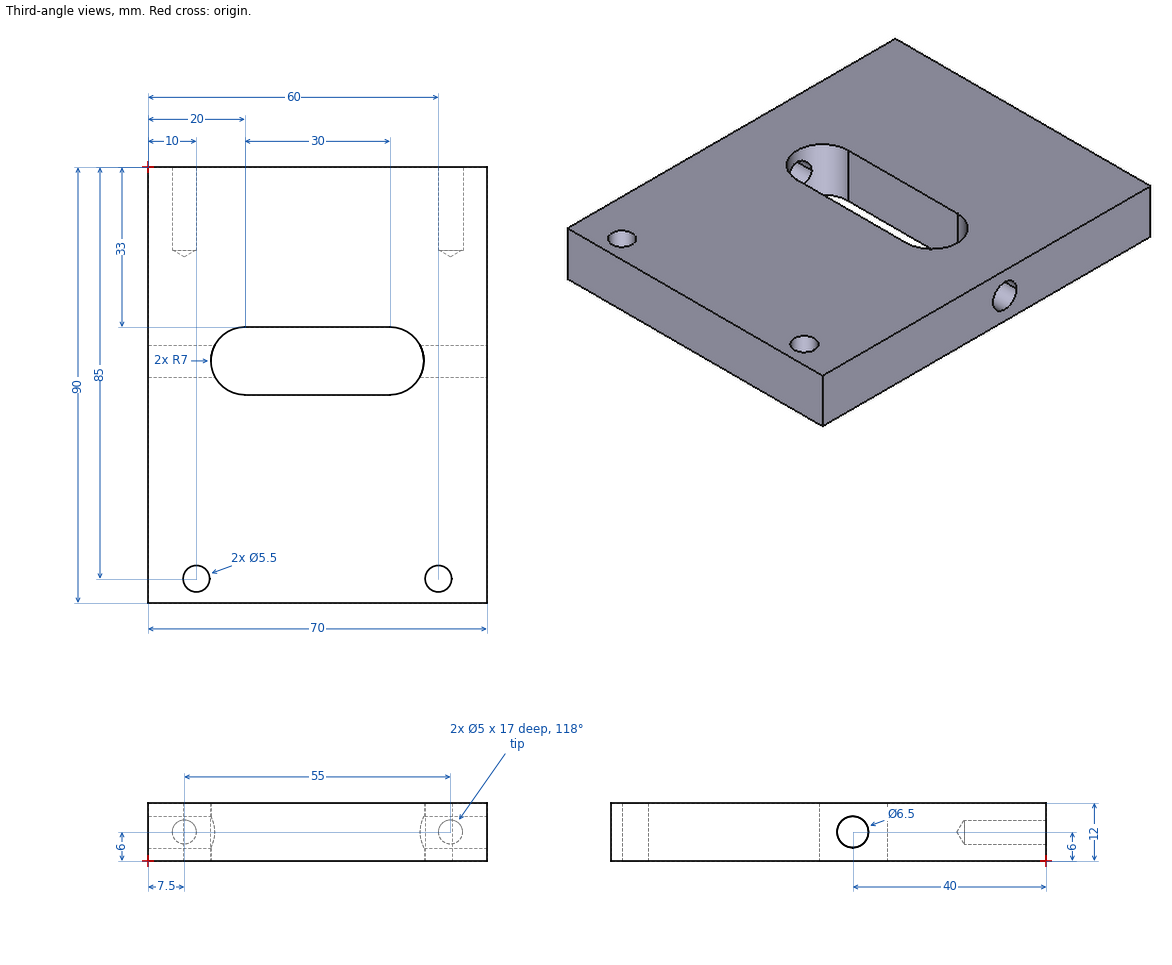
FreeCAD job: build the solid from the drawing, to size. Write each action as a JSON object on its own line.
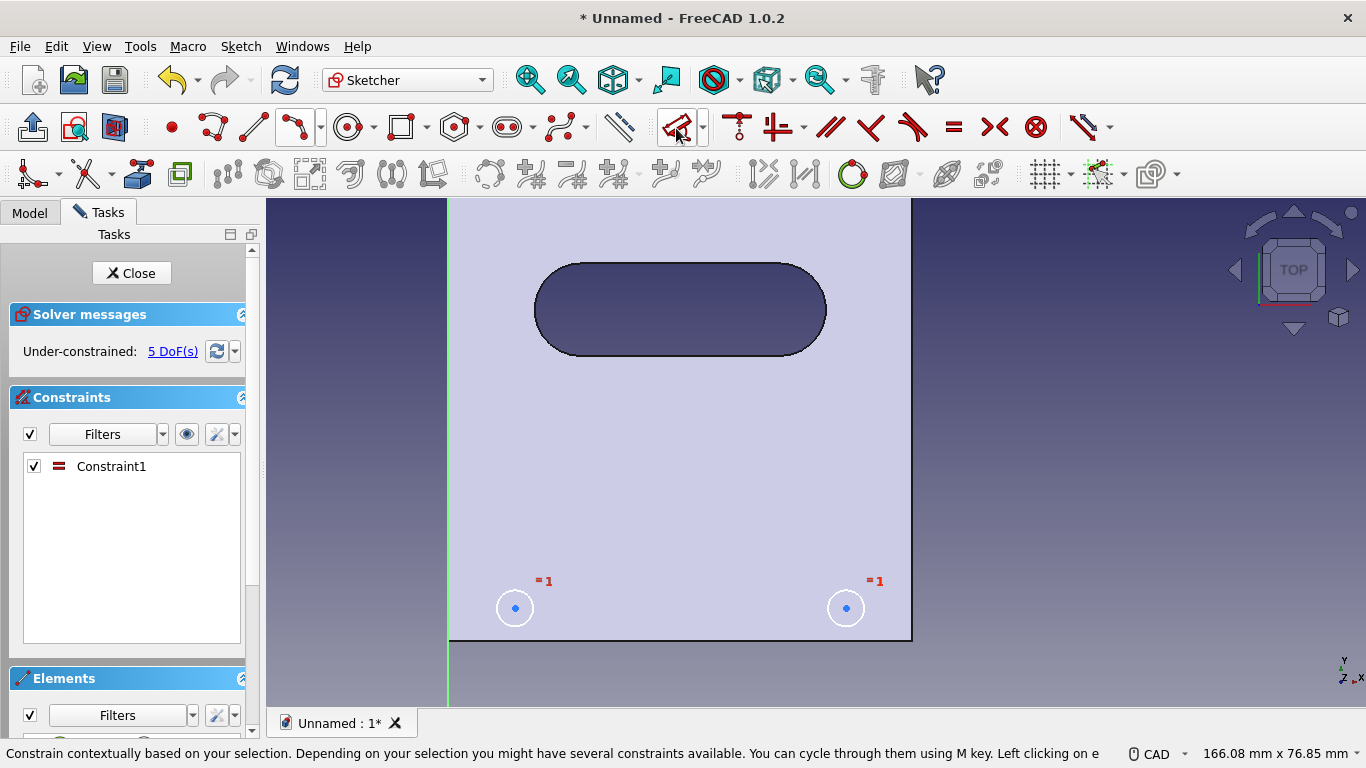
{"action": "left_click", "coordinate": [528, 596]}
{"action": "left_click", "coordinate": [551, 574]}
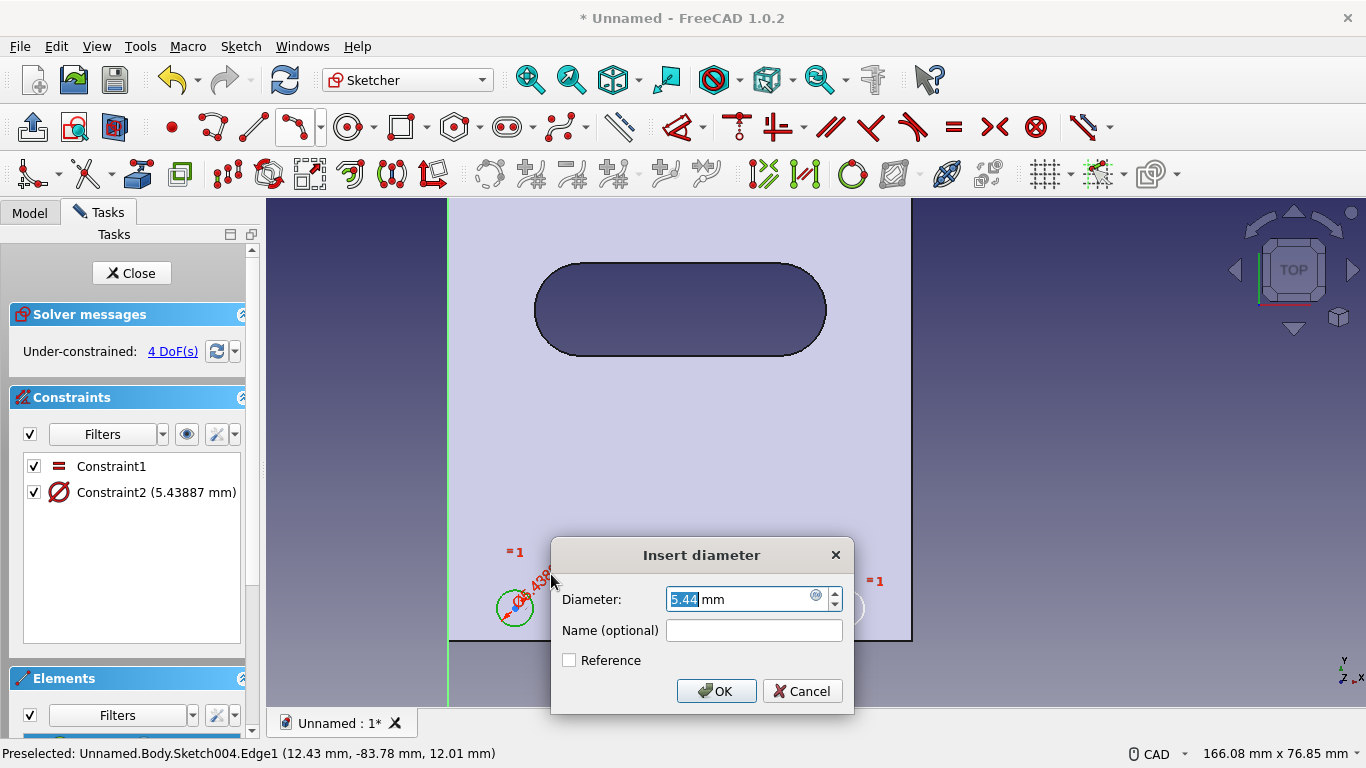
{"action": "type", "text": "5.5"}
{"action": "key", "text": "Return"}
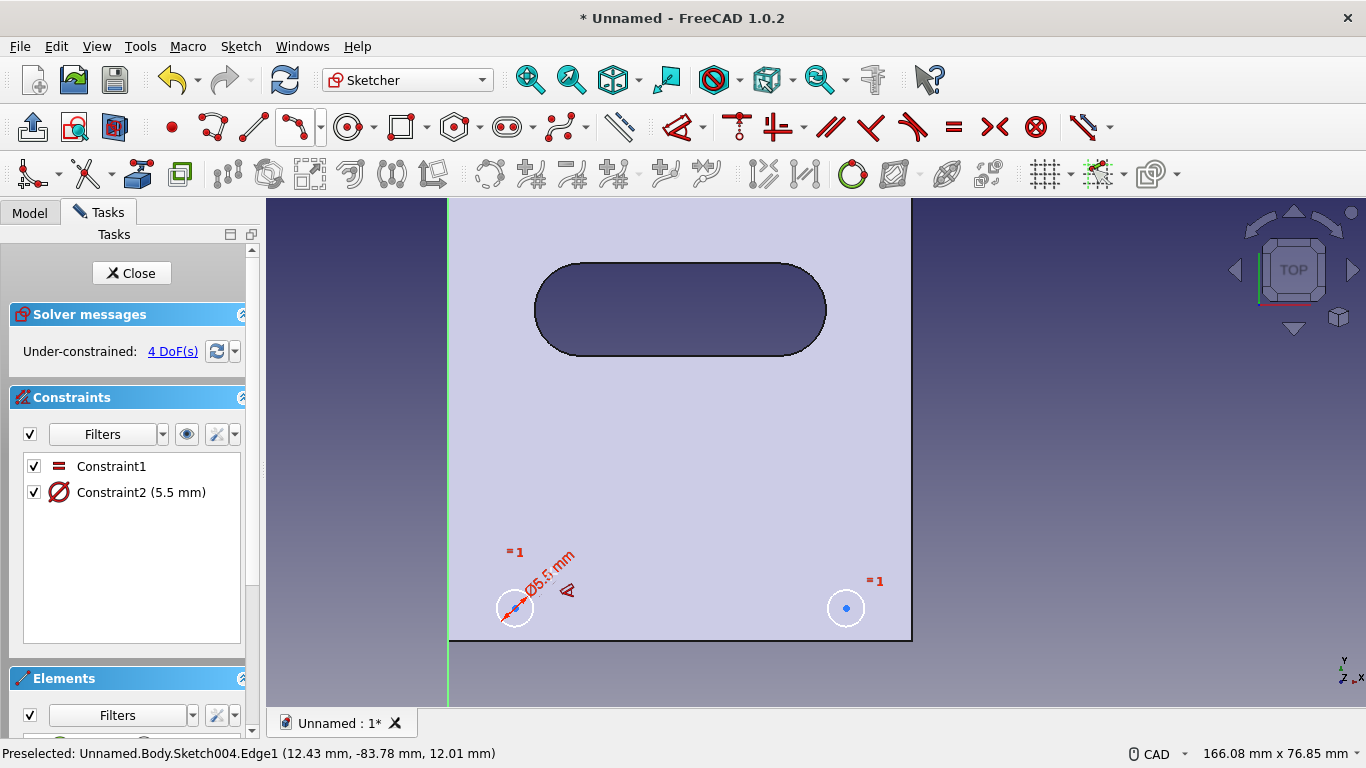
{"action": "left_click", "coordinate": [515, 608]}
{"action": "left_click", "coordinate": [482, 642]}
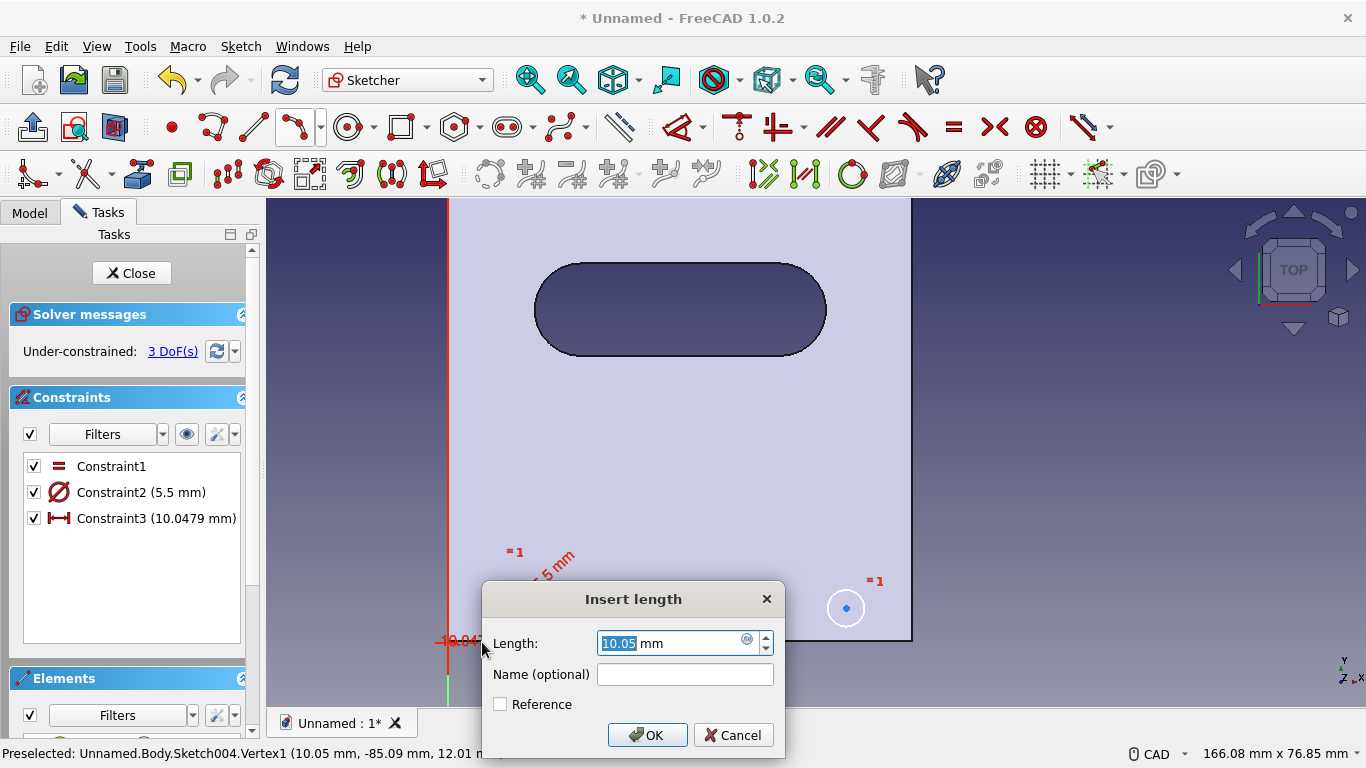
{"action": "type", "text": "10"}
{"action": "key", "text": "Return"}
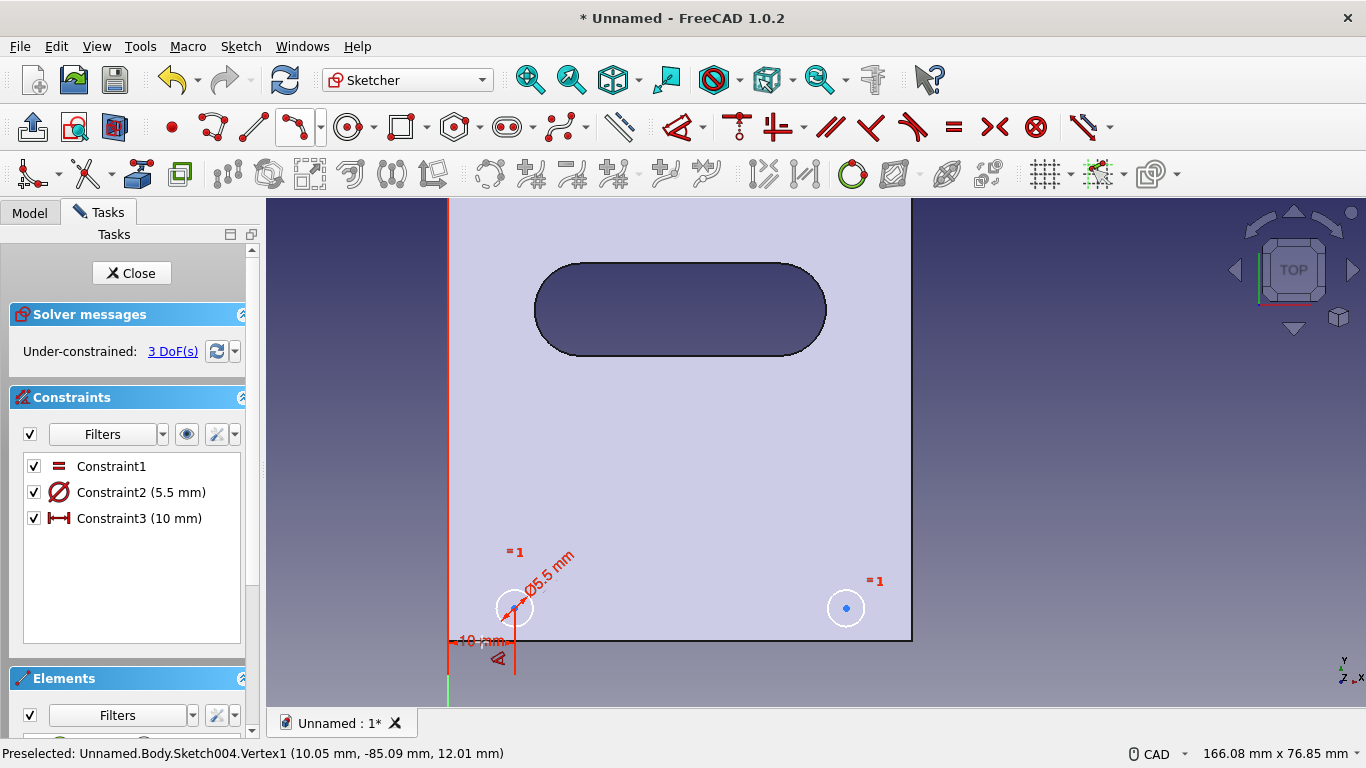
{"action": "left_click", "coordinate": [515, 608]}
{"action": "left_click", "coordinate": [414, 417]}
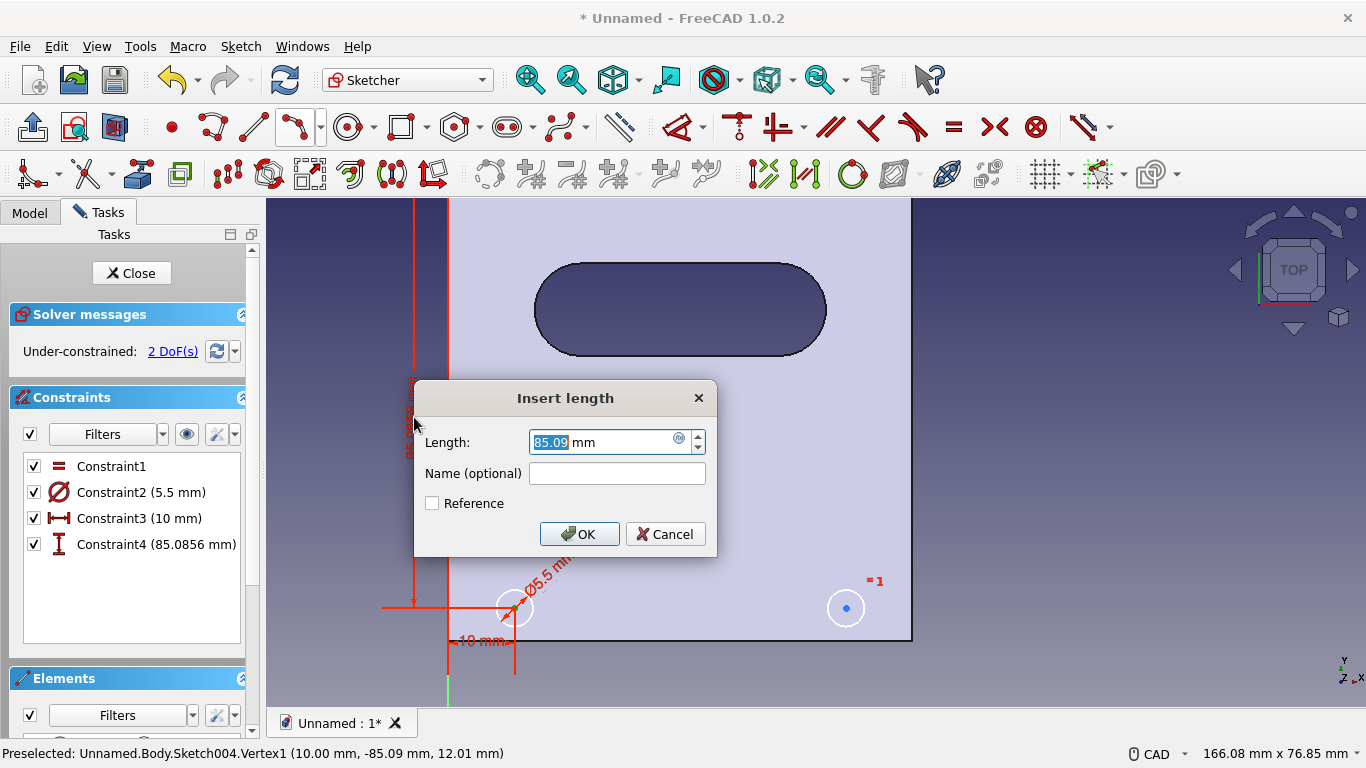
{"action": "type", "text": "85"}
{"action": "key", "text": "Return"}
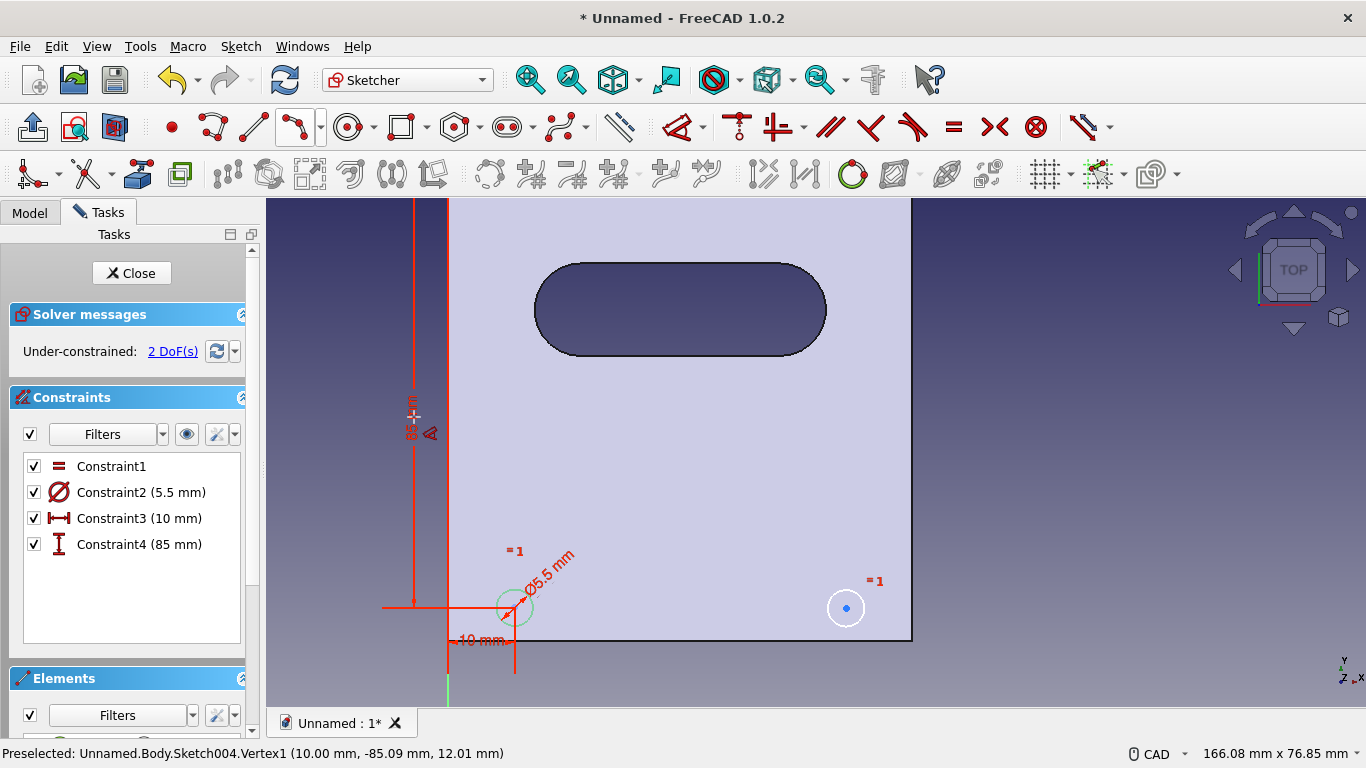
{"action": "left_click", "coordinate": [846, 608]}
{"action": "left_click", "coordinate": [647, 642]}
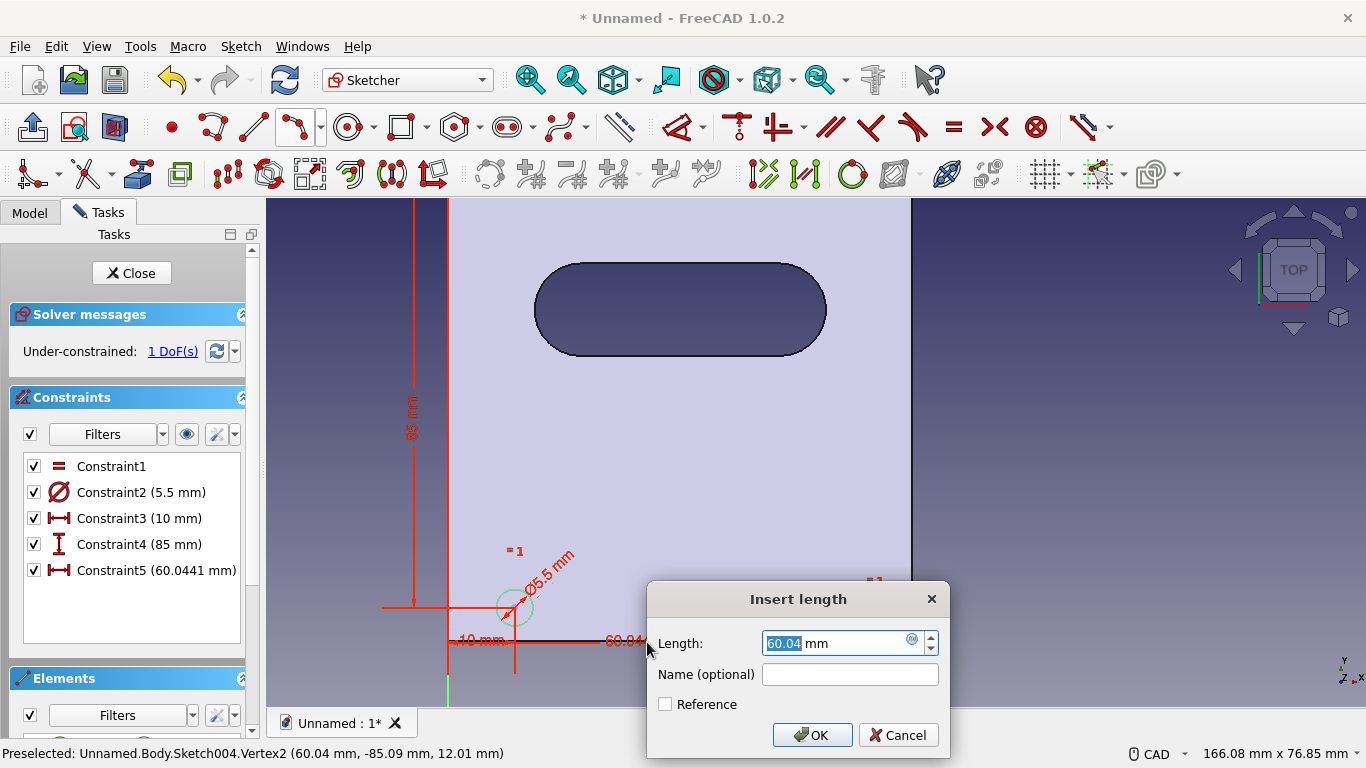
{"action": "type", "text": "60"}
{"action": "key", "text": "Return"}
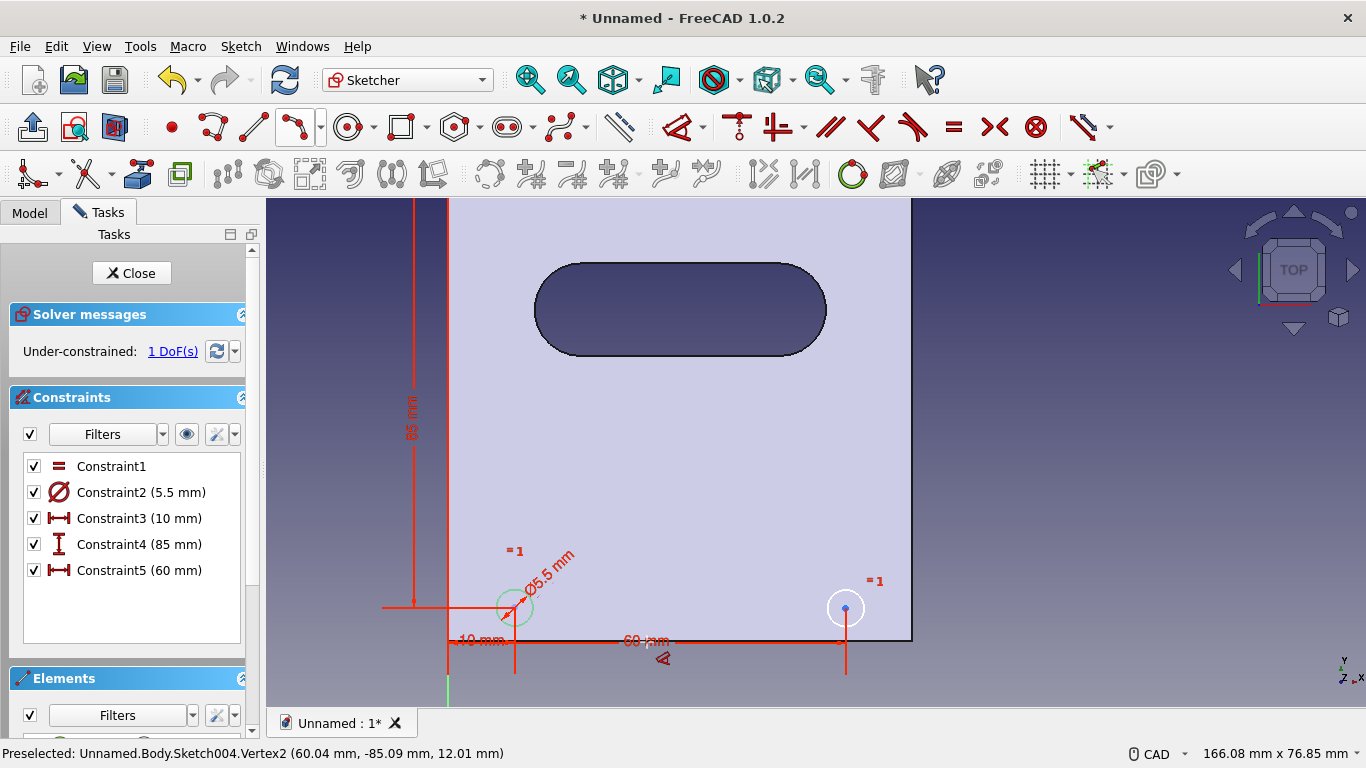
{"action": "left_click", "coordinate": [846, 608]}
{"action": "left_click", "coordinate": [414, 329]}